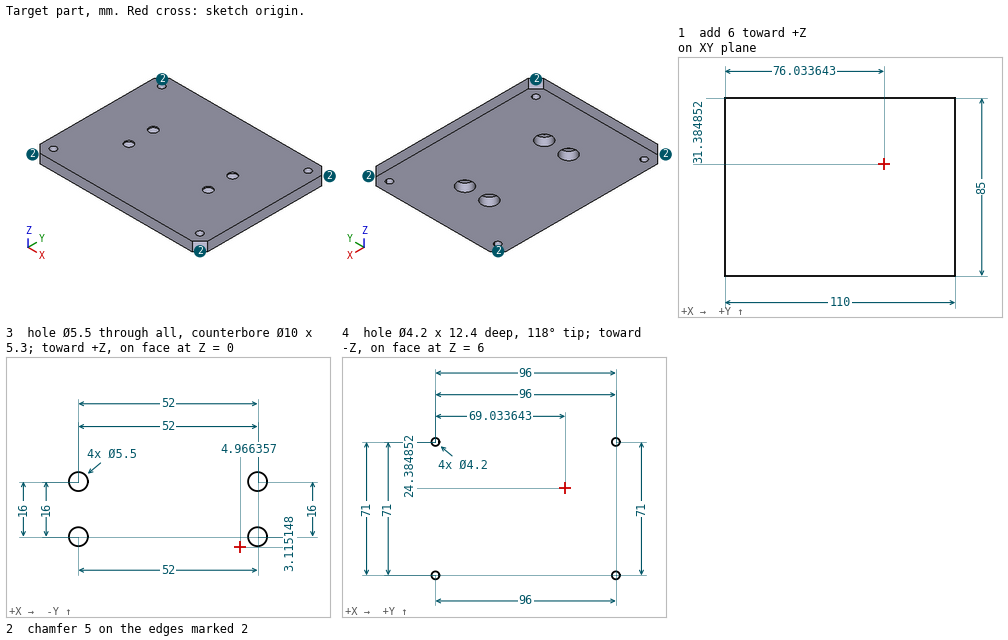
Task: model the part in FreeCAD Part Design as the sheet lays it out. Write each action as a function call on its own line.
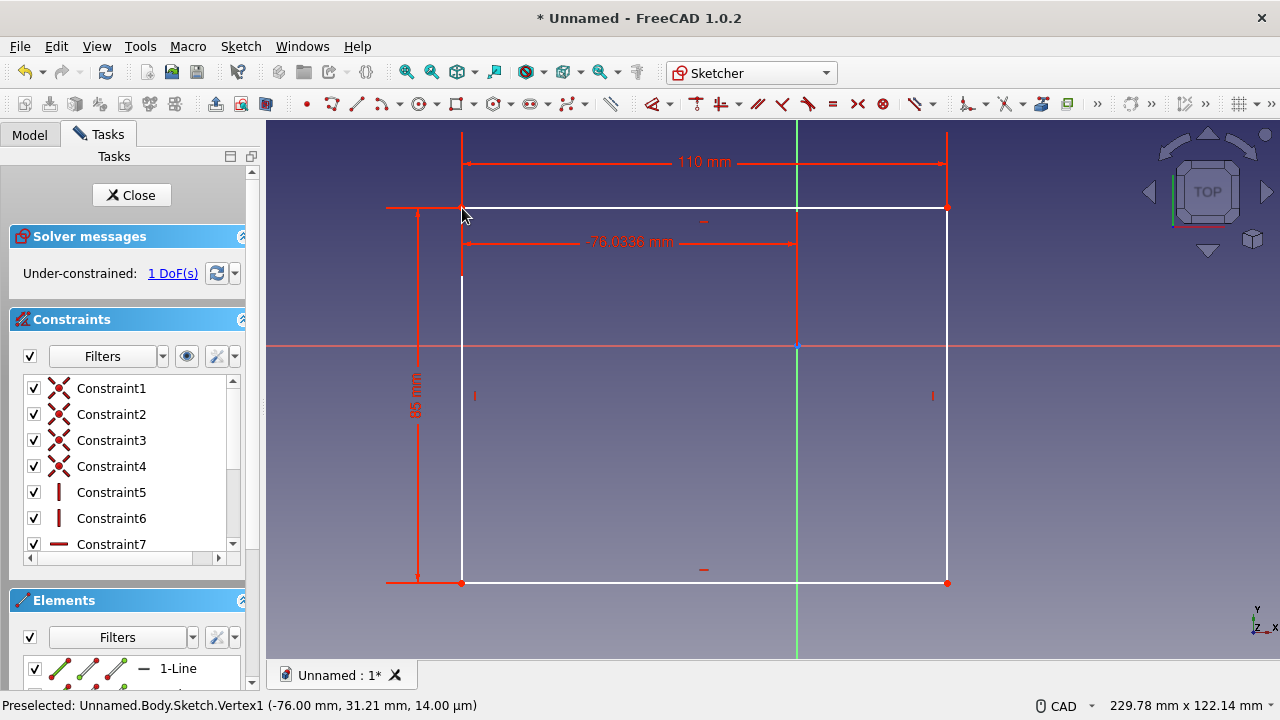
click(462, 208)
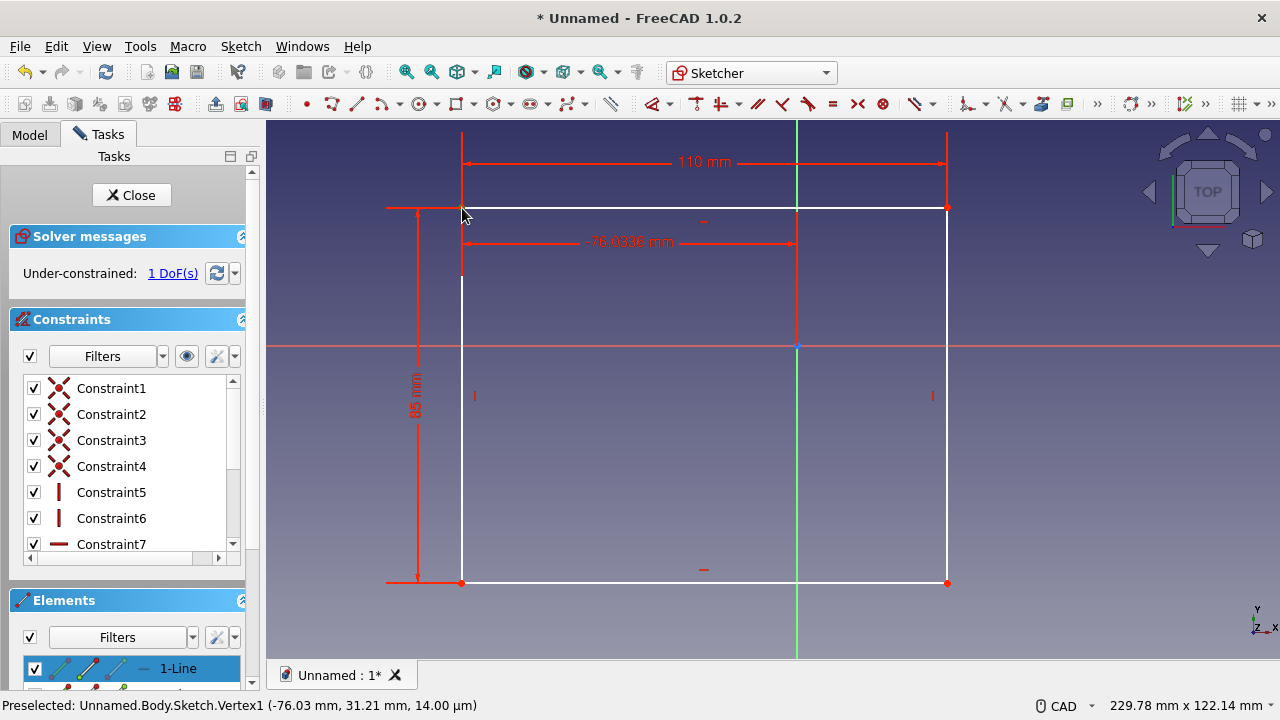
key(i)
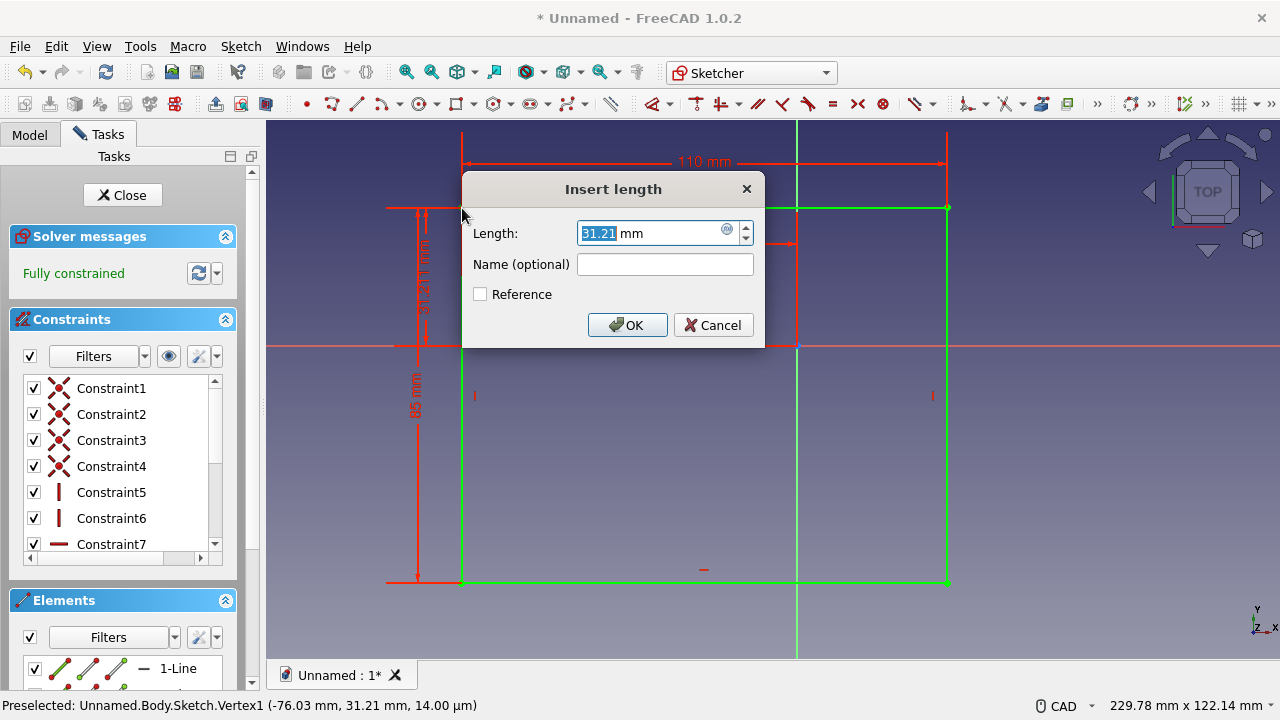
text(31.384852)
key(Return)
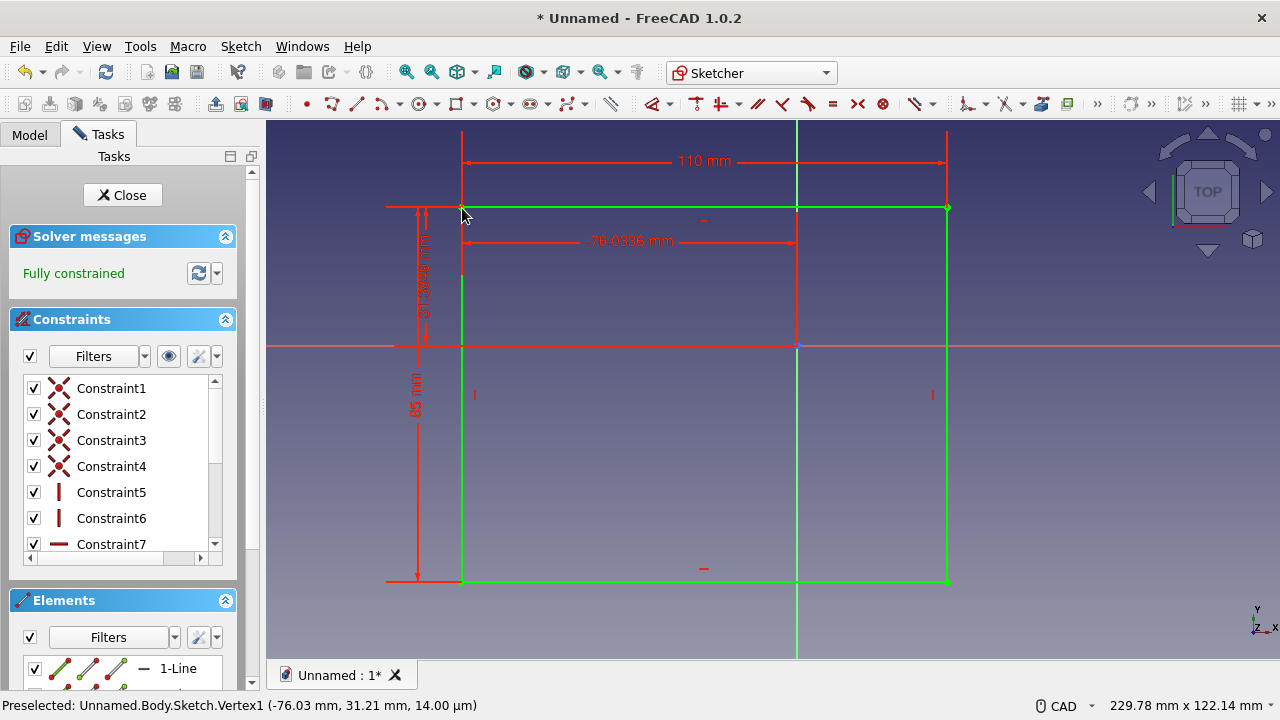
click(123, 195)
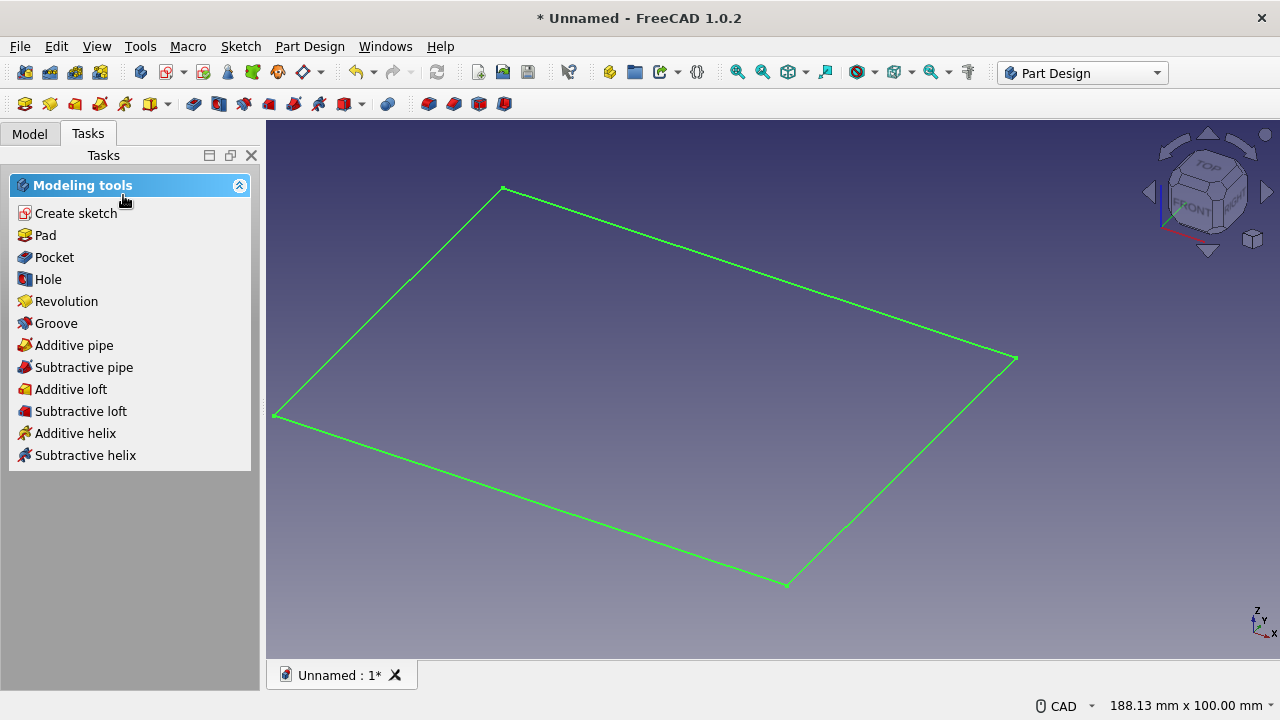
click(25, 104)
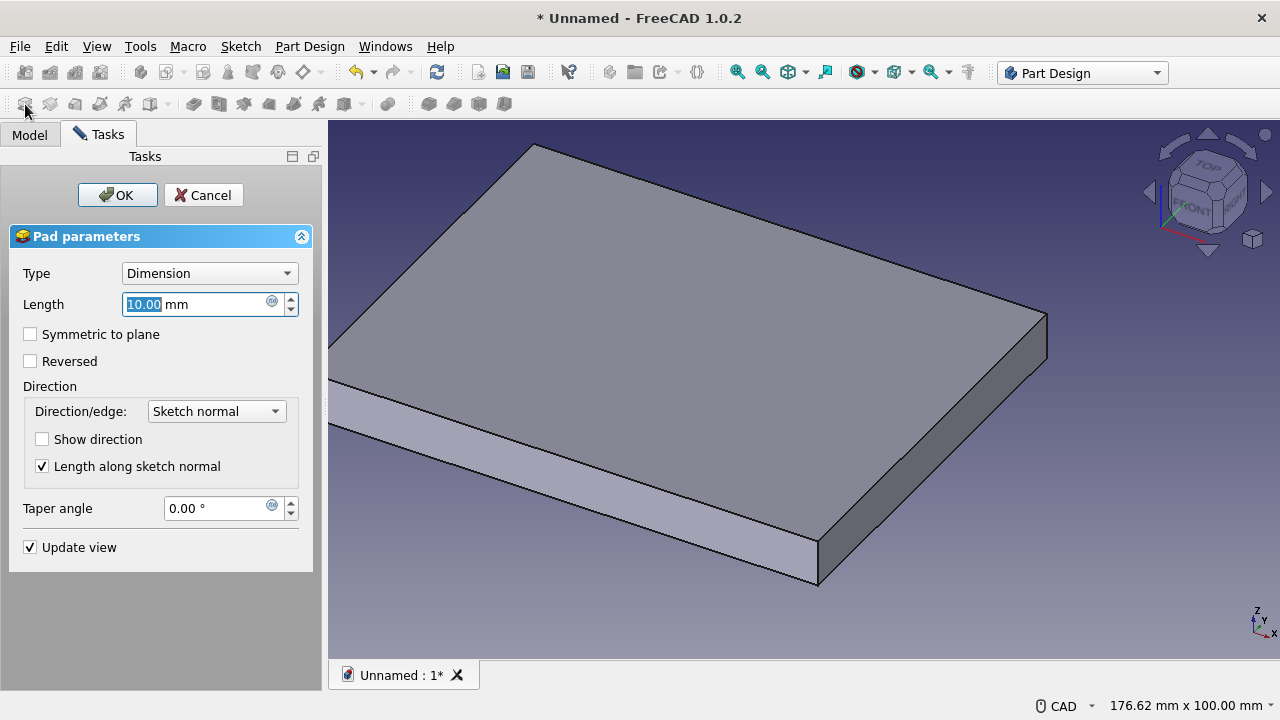
text(6)
key(Tab)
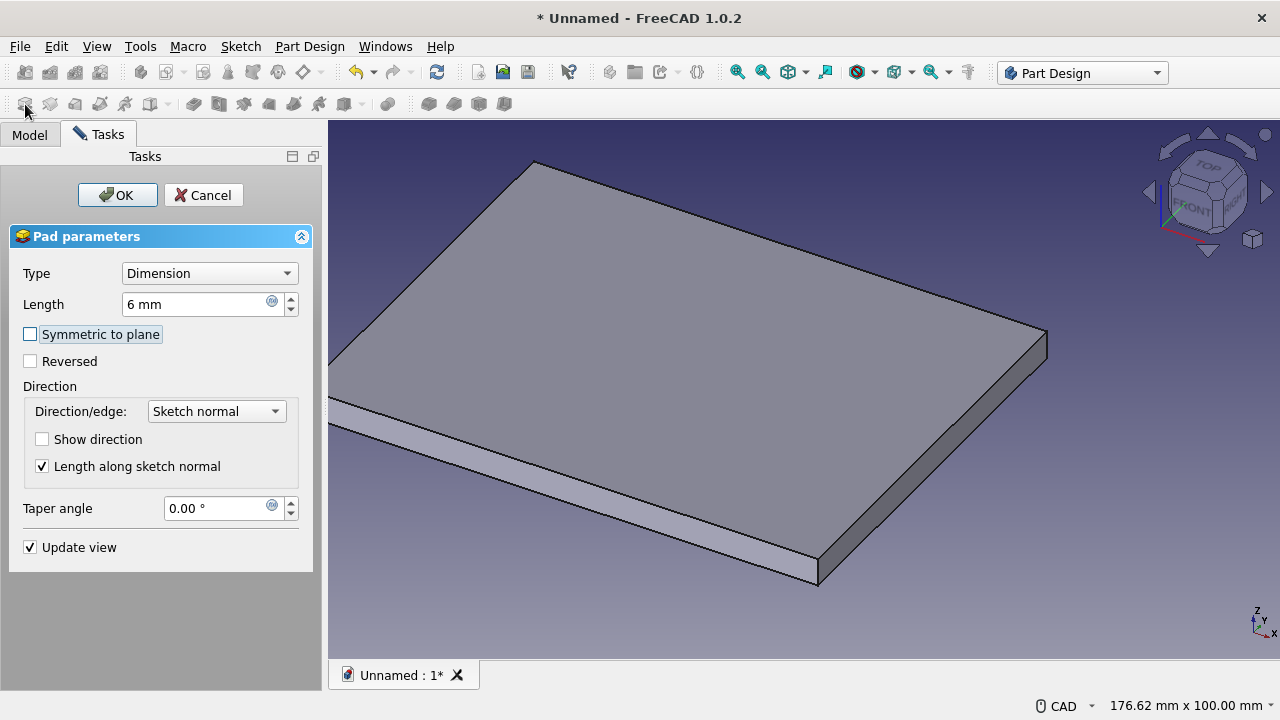
click(118, 195)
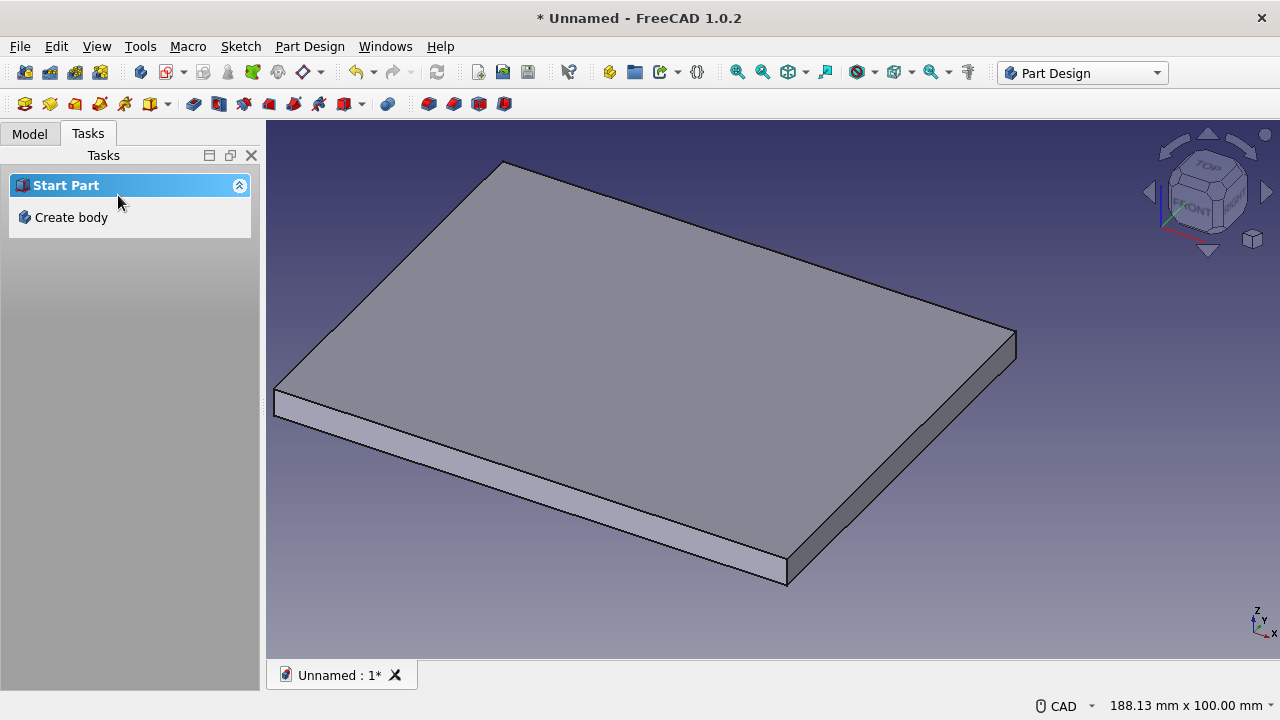
click(787, 571)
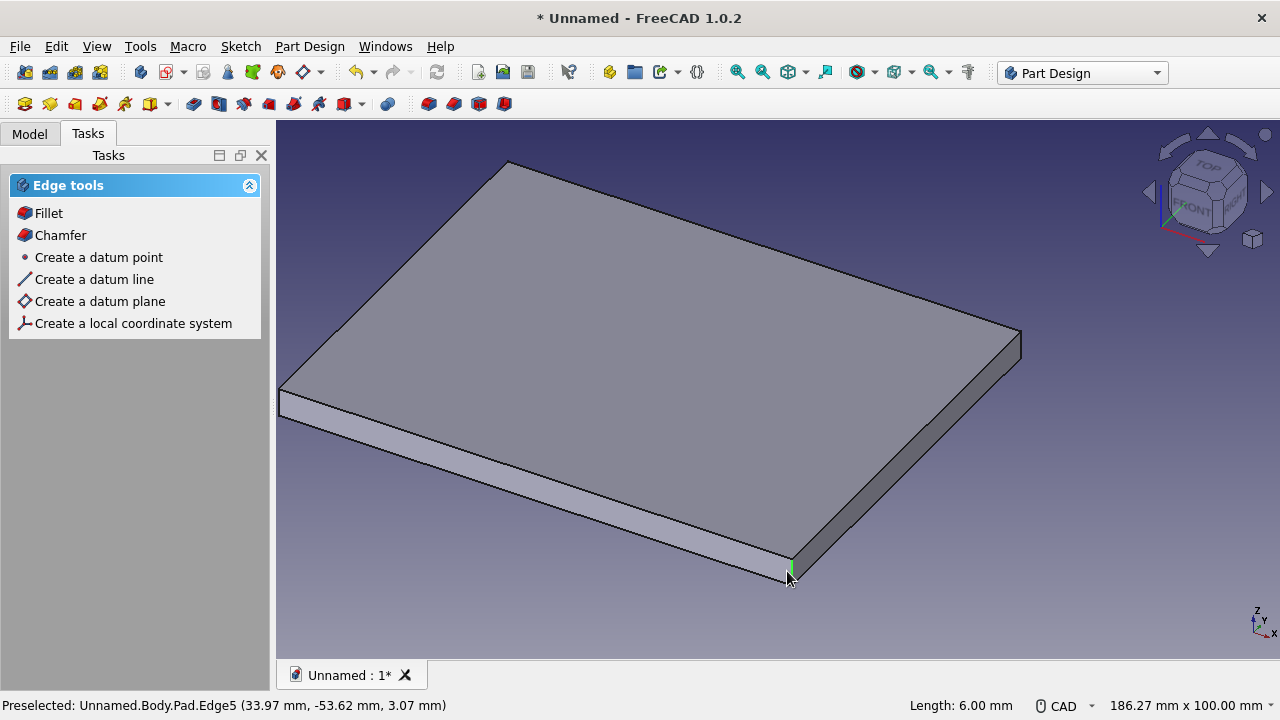
key(0)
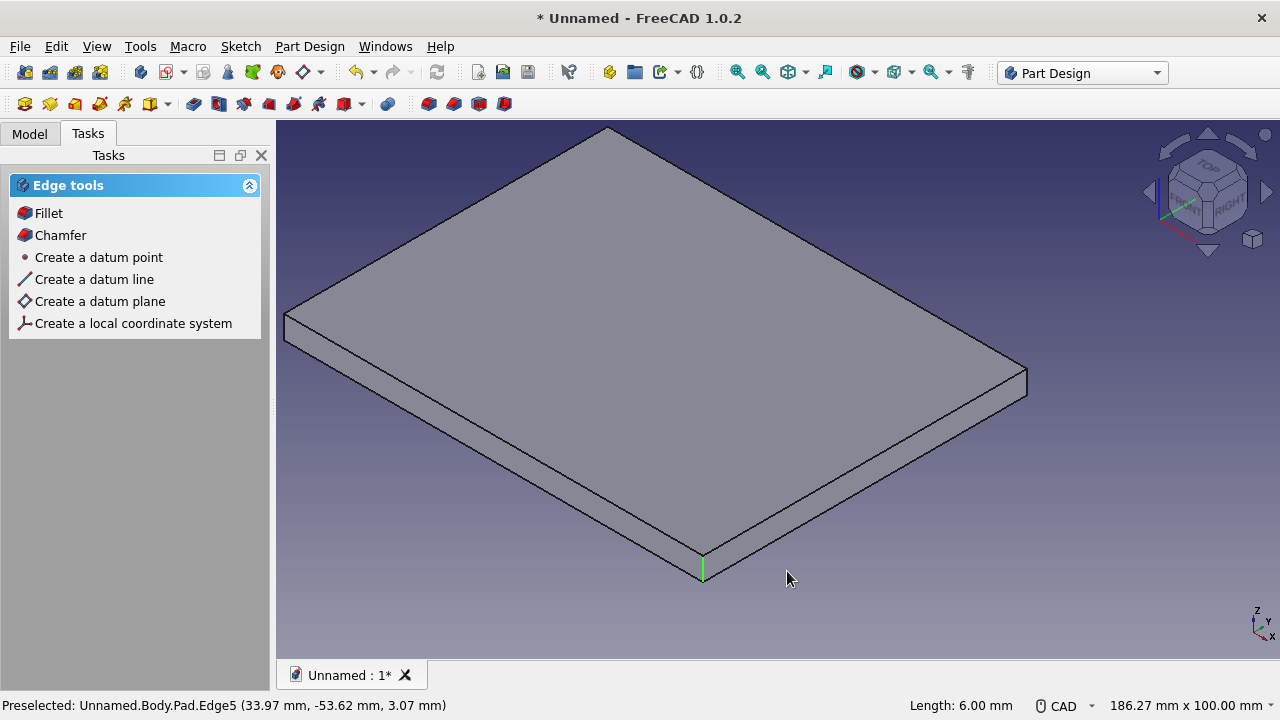
key(2)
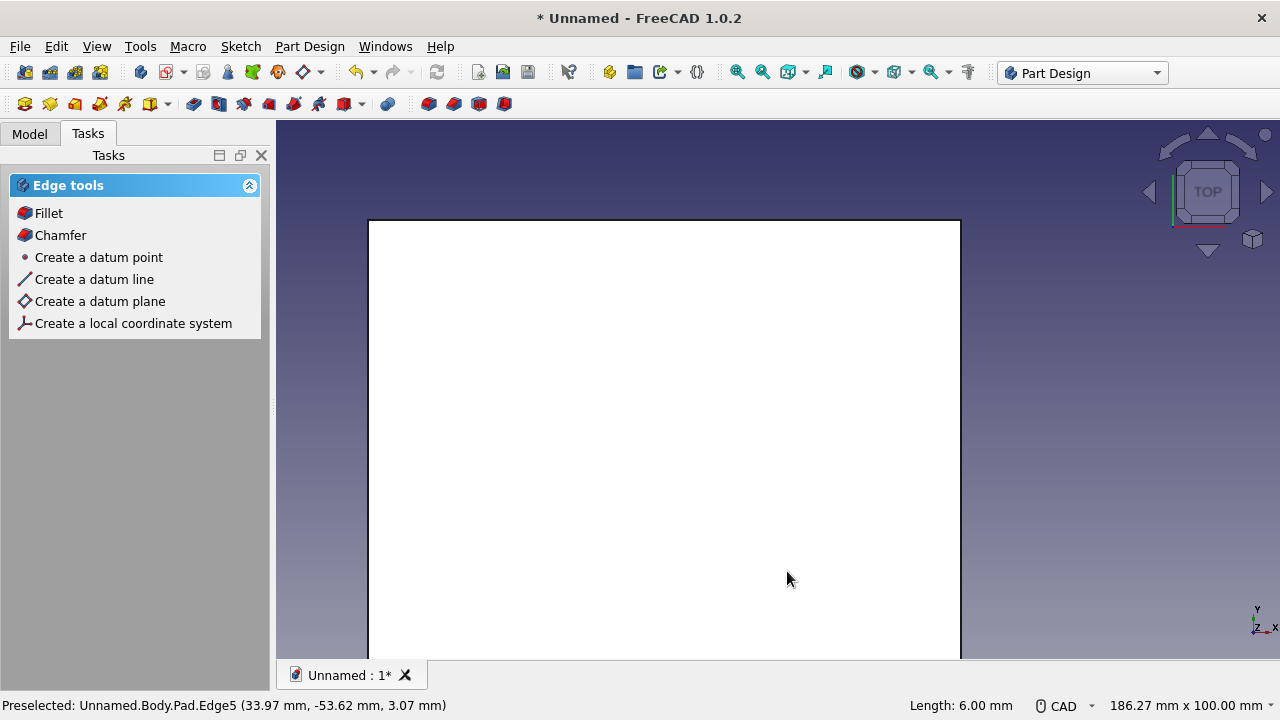
click(738, 72)